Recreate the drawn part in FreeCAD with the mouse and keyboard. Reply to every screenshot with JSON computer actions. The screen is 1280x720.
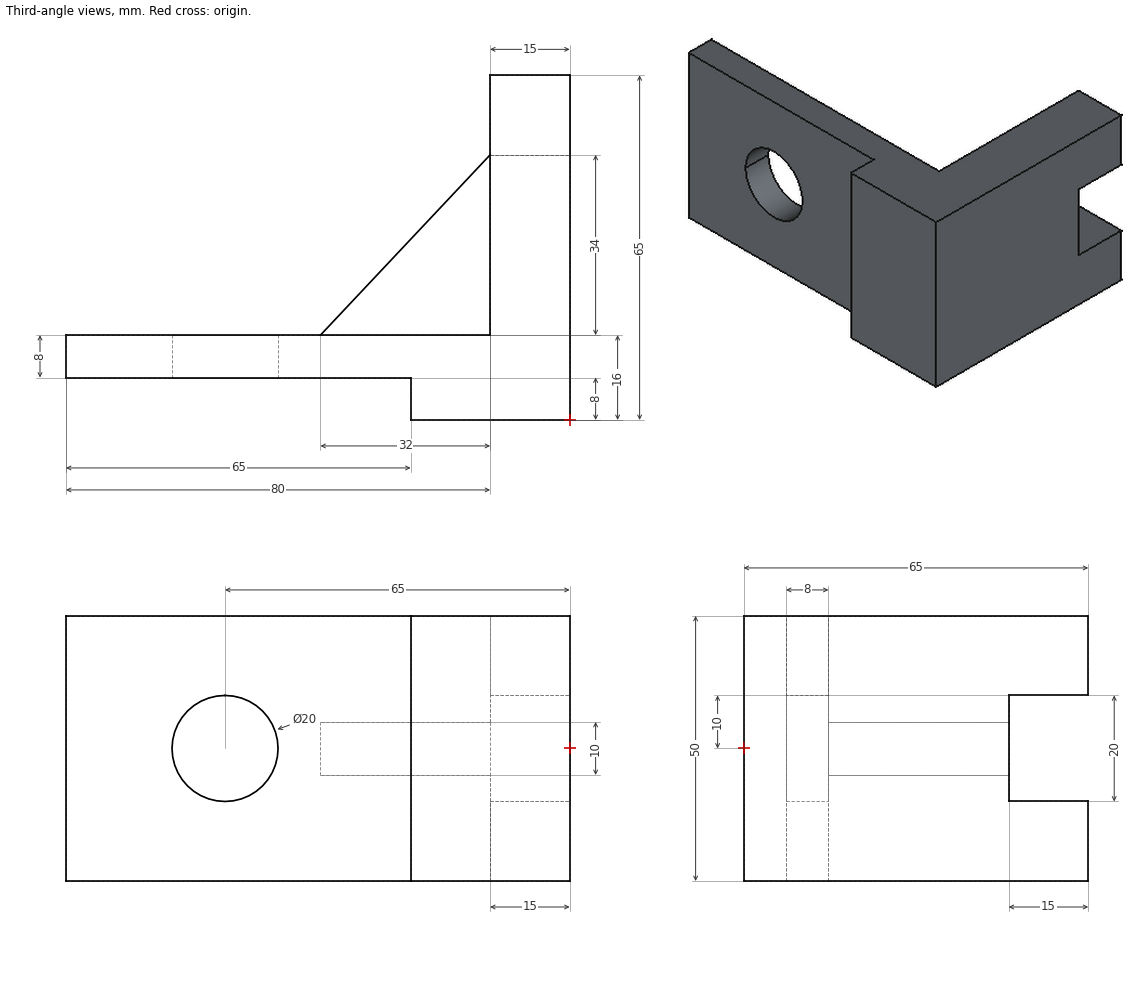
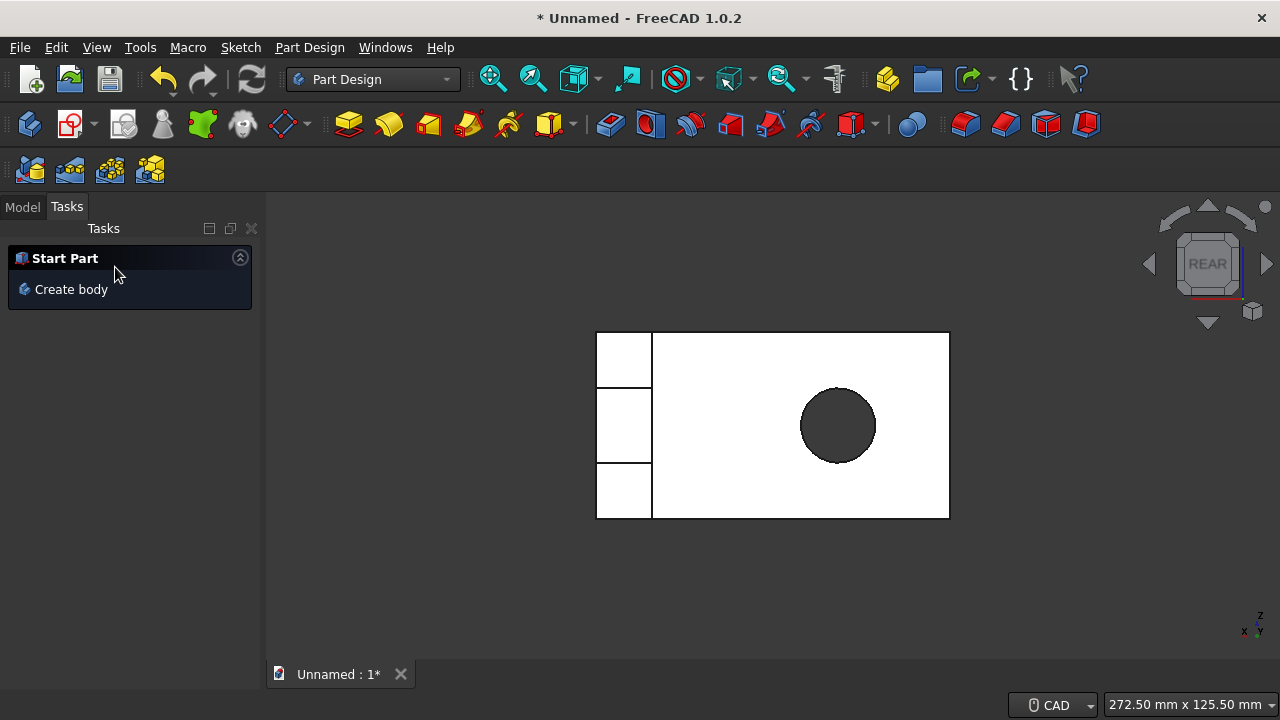
{"action": "key", "text": "v f"}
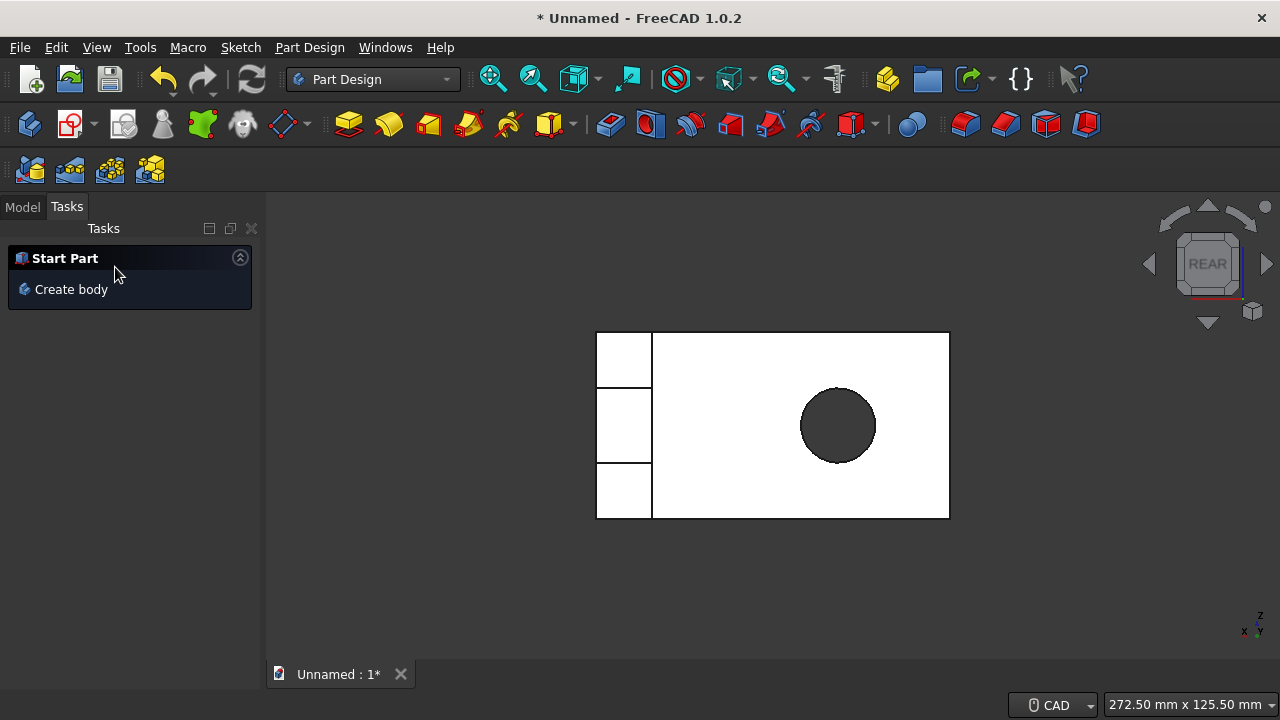
{"action": "left_click", "coordinate": [70, 124]}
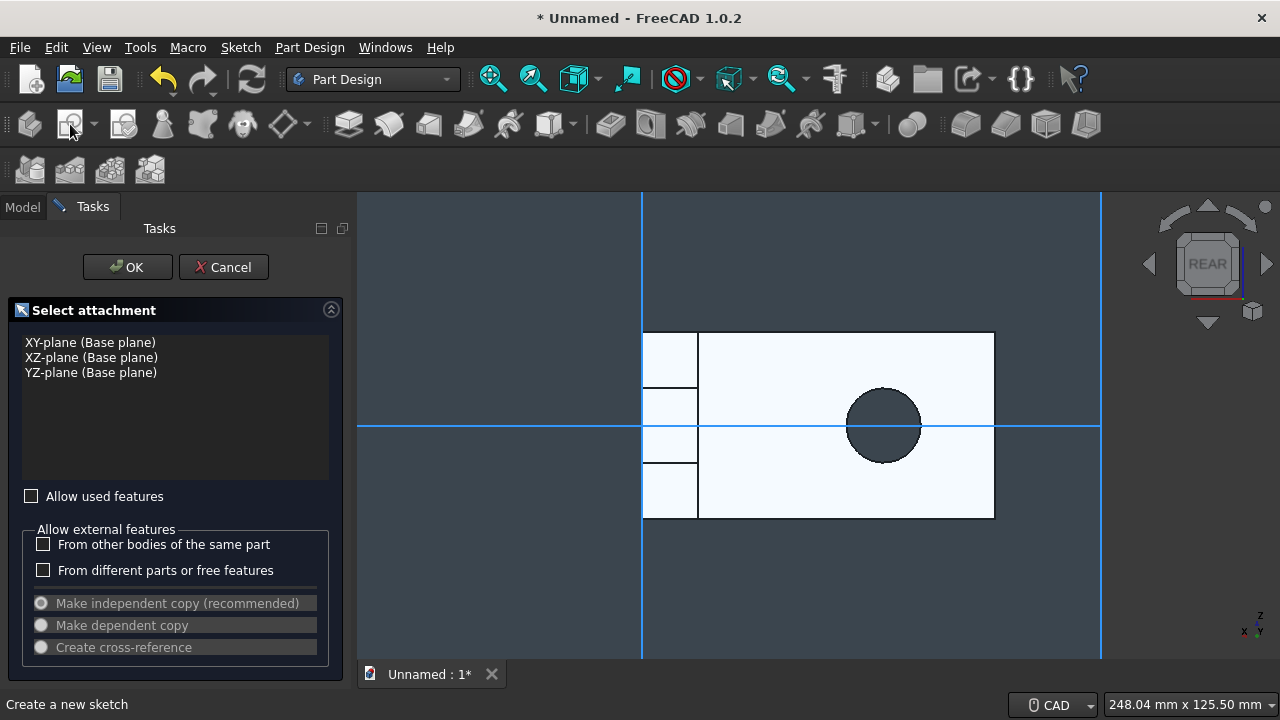
{"action": "left_click", "coordinate": [82, 342]}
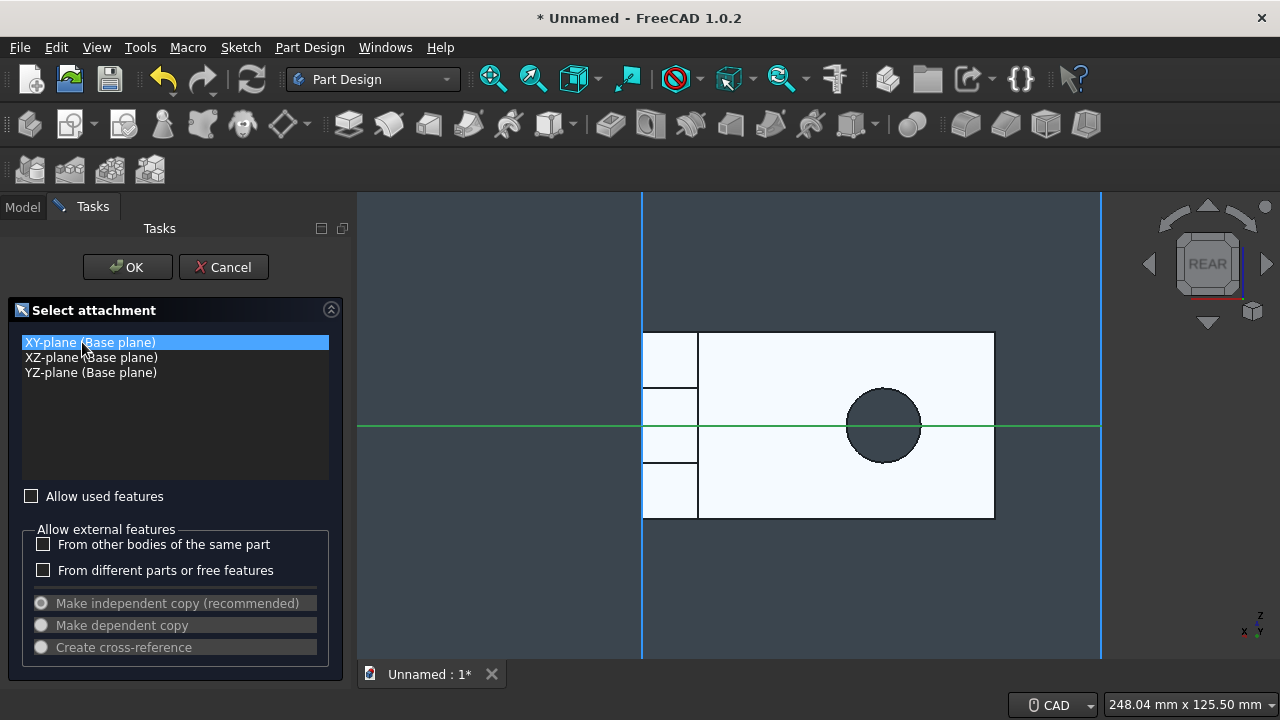
{"action": "left_click", "coordinate": [128, 267]}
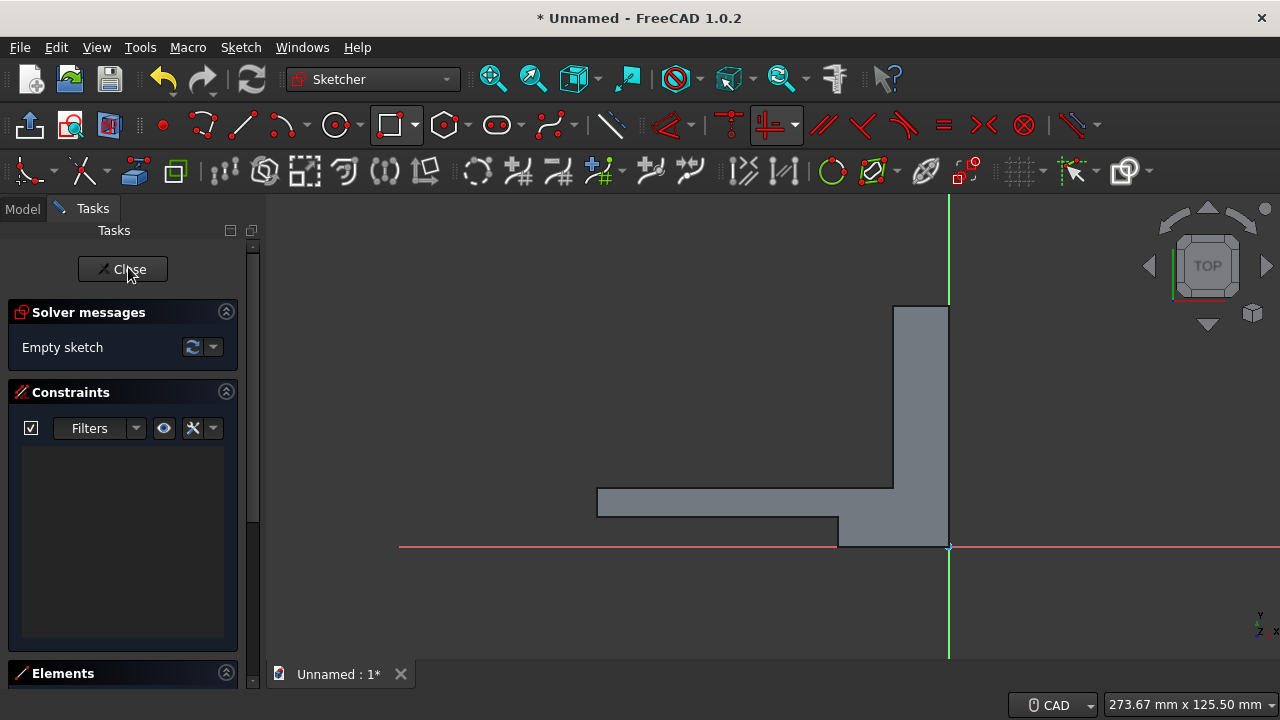
{"action": "key", "text": "q s"}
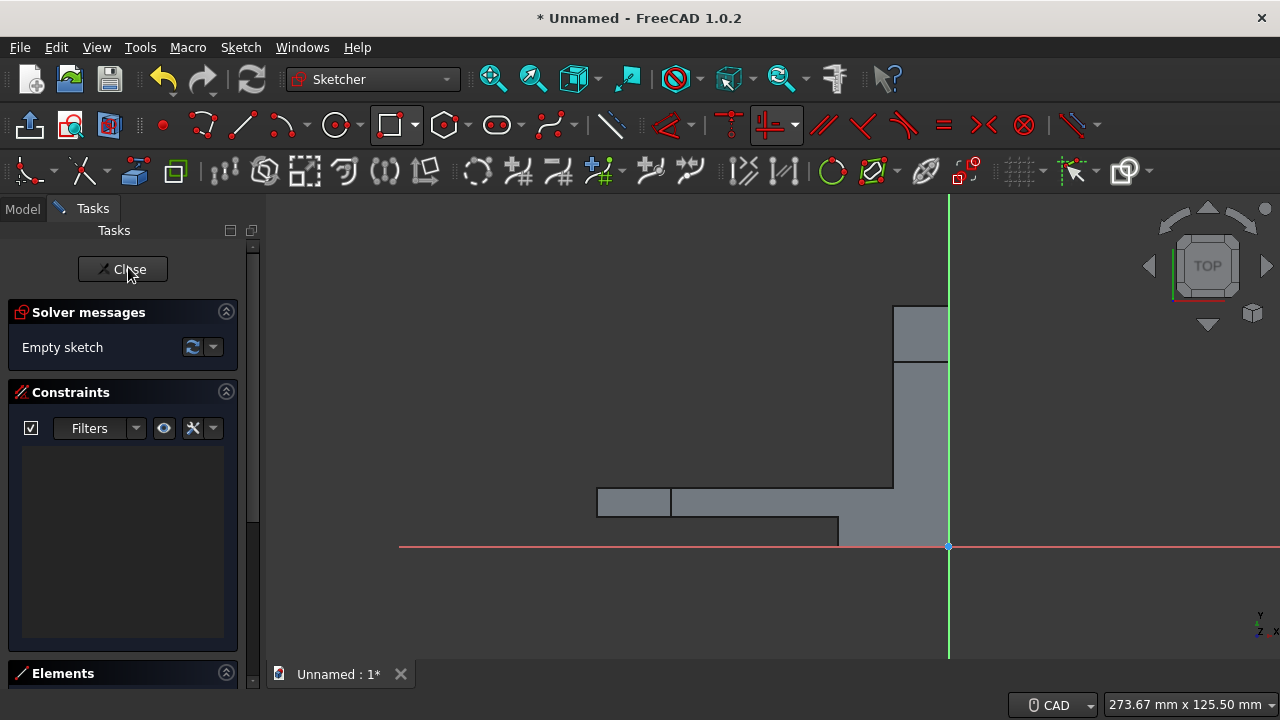
{"action": "scroll", "coordinate": [1115, 511], "scroll_direction": "up", "scroll_amount": 2}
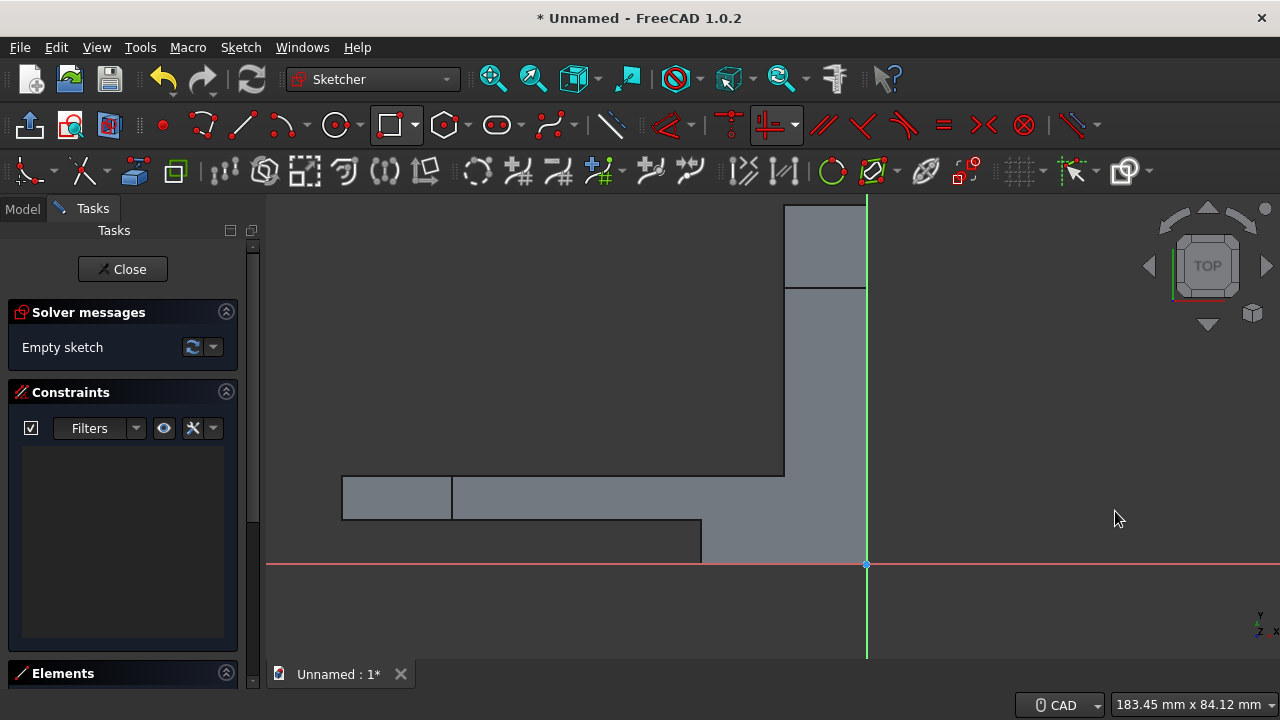
{"action": "left_click", "coordinate": [204, 126]}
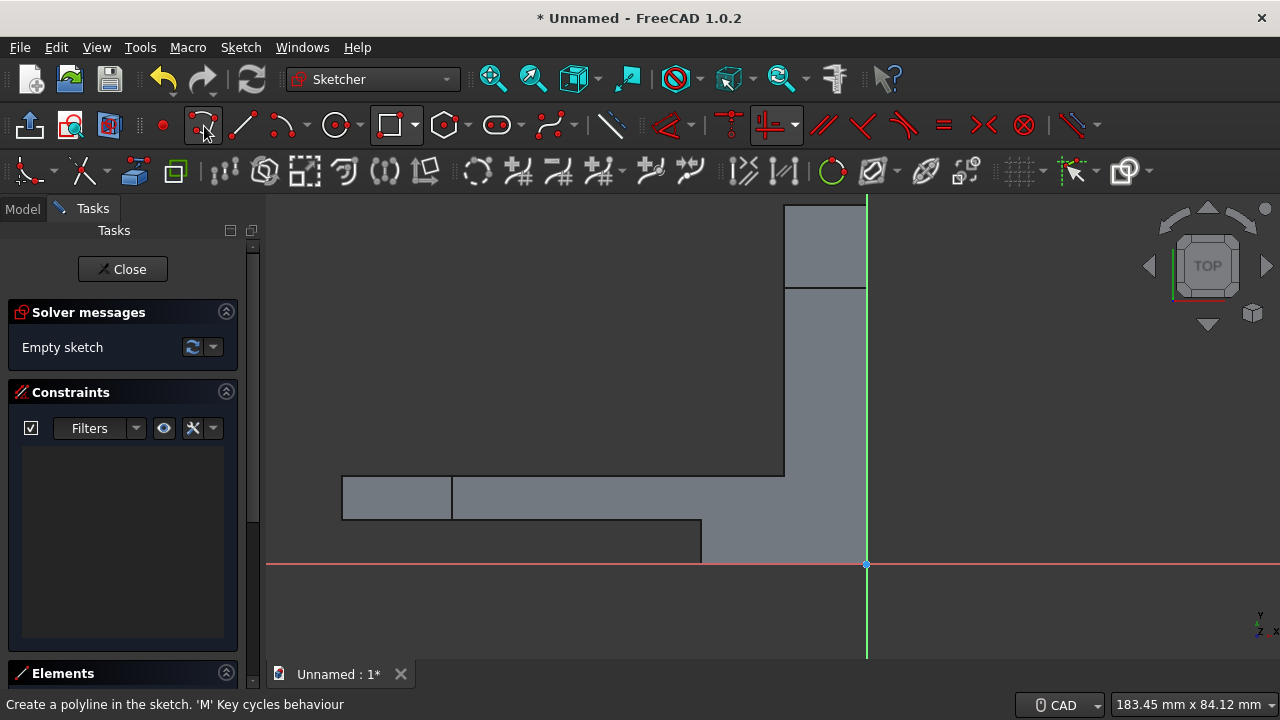
{"action": "left_click", "coordinate": [784, 476]}
{"action": "left_click", "coordinate": [784, 288]}
{"action": "left_click", "coordinate": [607, 476]}
{"action": "left_click", "coordinate": [784, 477]}
{"action": "key", "text": "Escape"}
{"action": "key", "text": "Escape"}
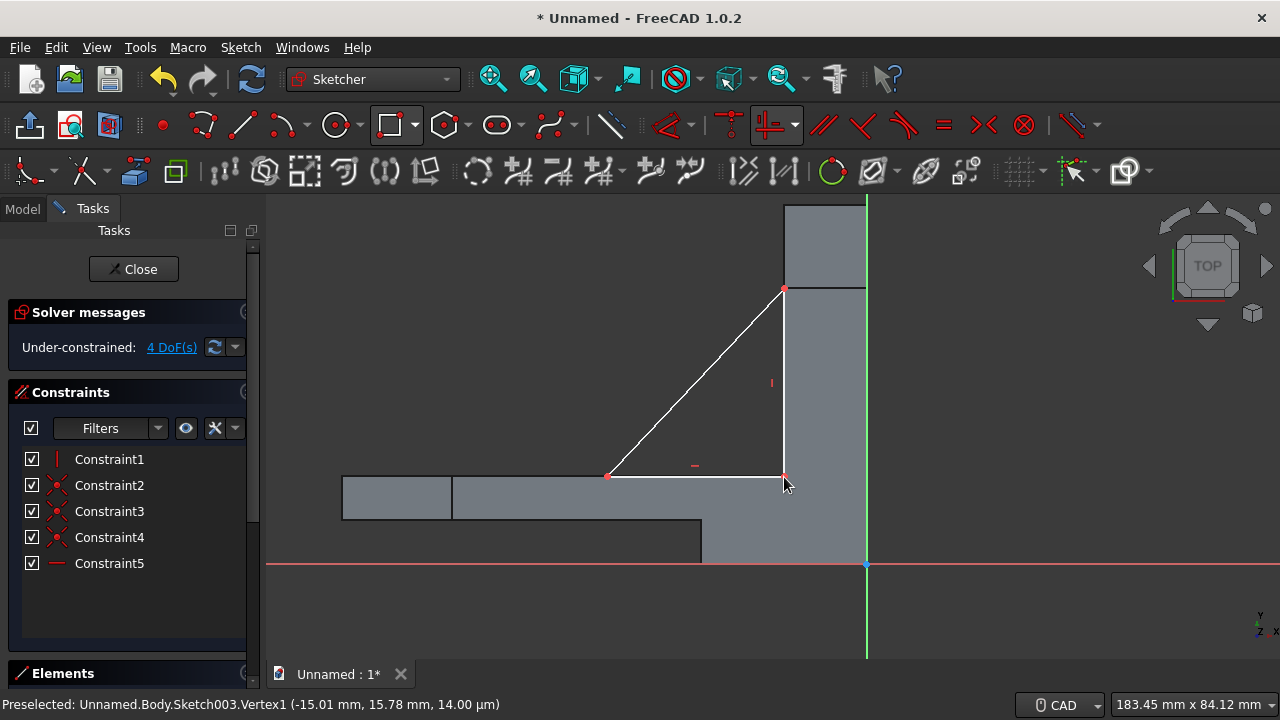
{"action": "key", "text": "d"}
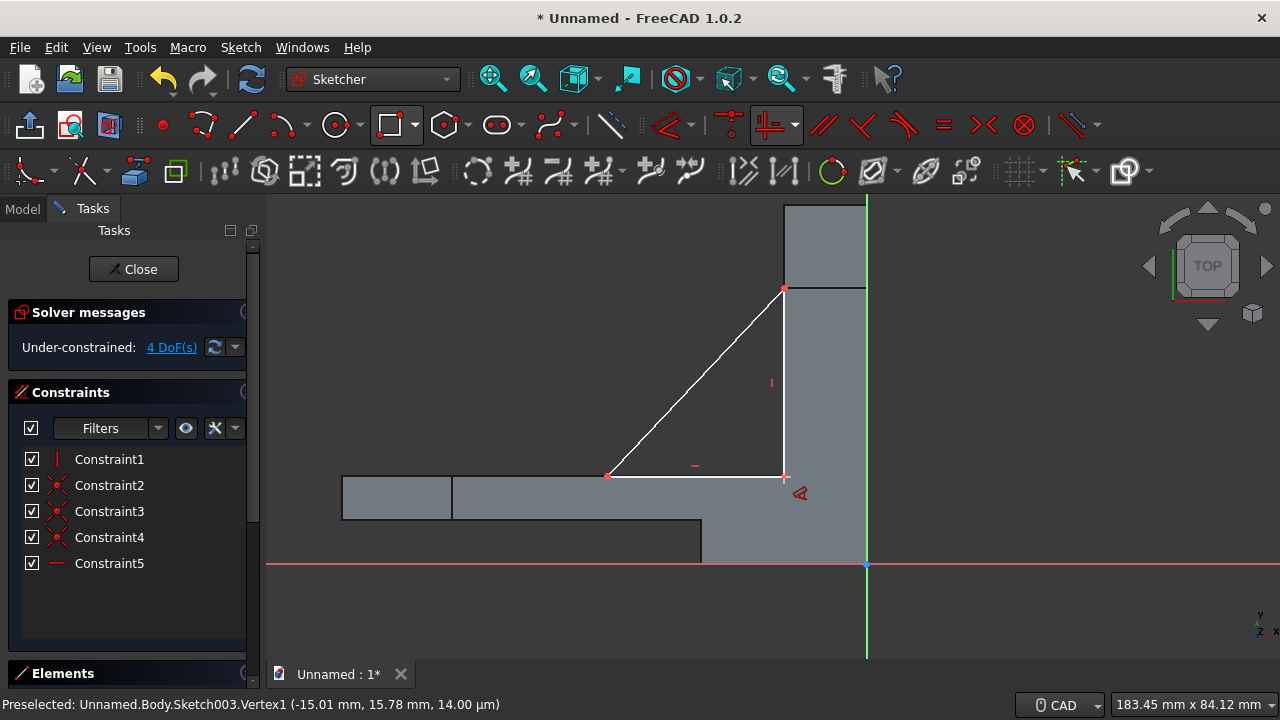
{"action": "left_click", "coordinate": [784, 421]}
{"action": "left_click", "coordinate": [818, 383]}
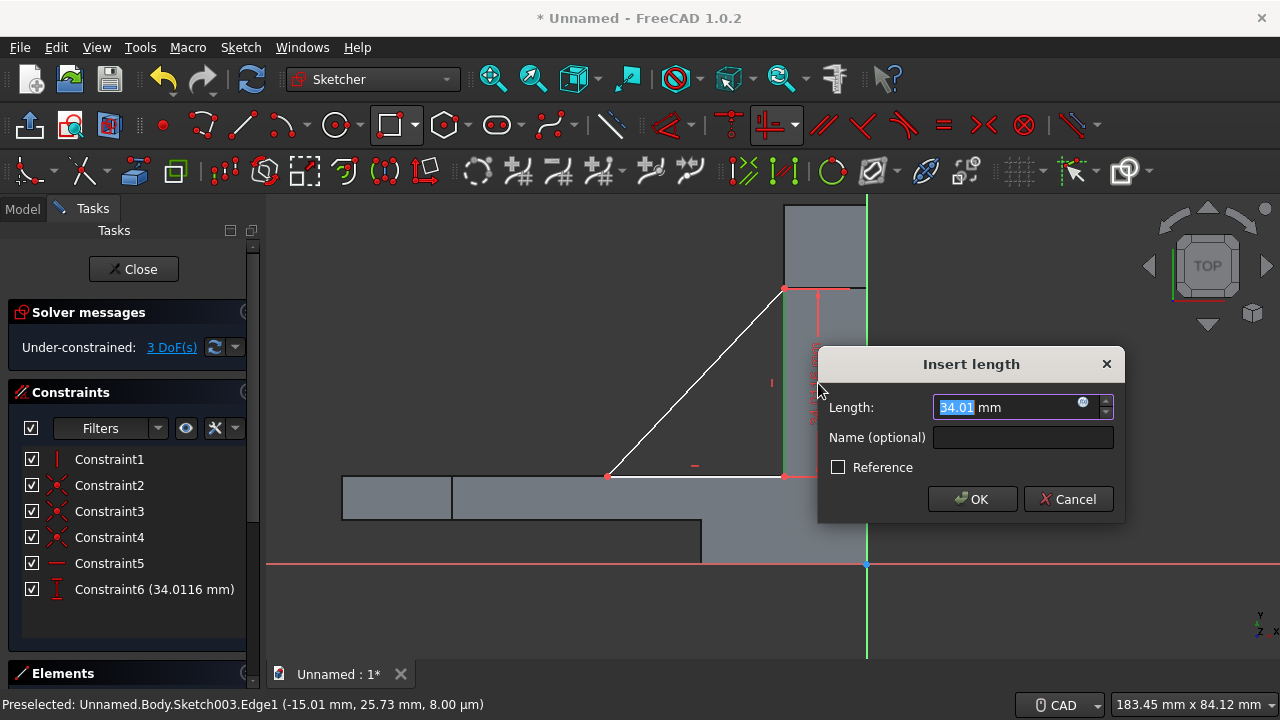
{"action": "type", "text": "34"}
{"action": "key", "text": "Return"}